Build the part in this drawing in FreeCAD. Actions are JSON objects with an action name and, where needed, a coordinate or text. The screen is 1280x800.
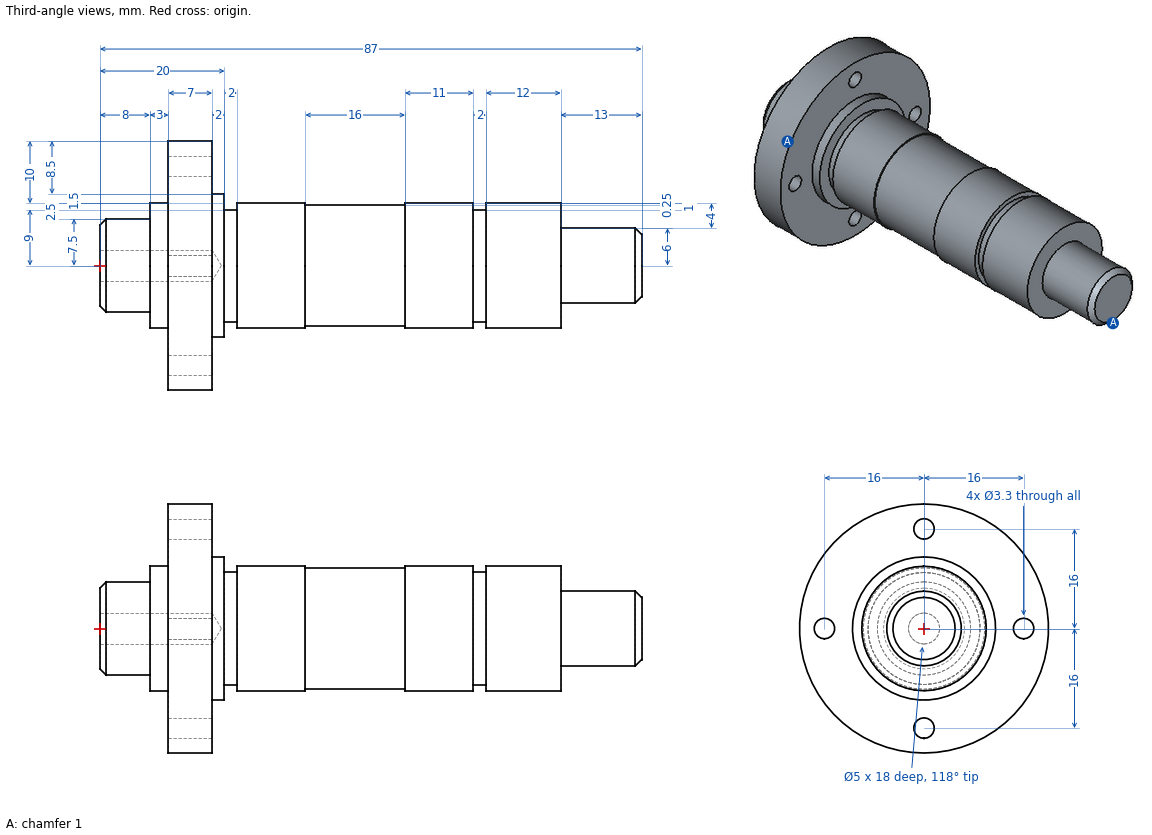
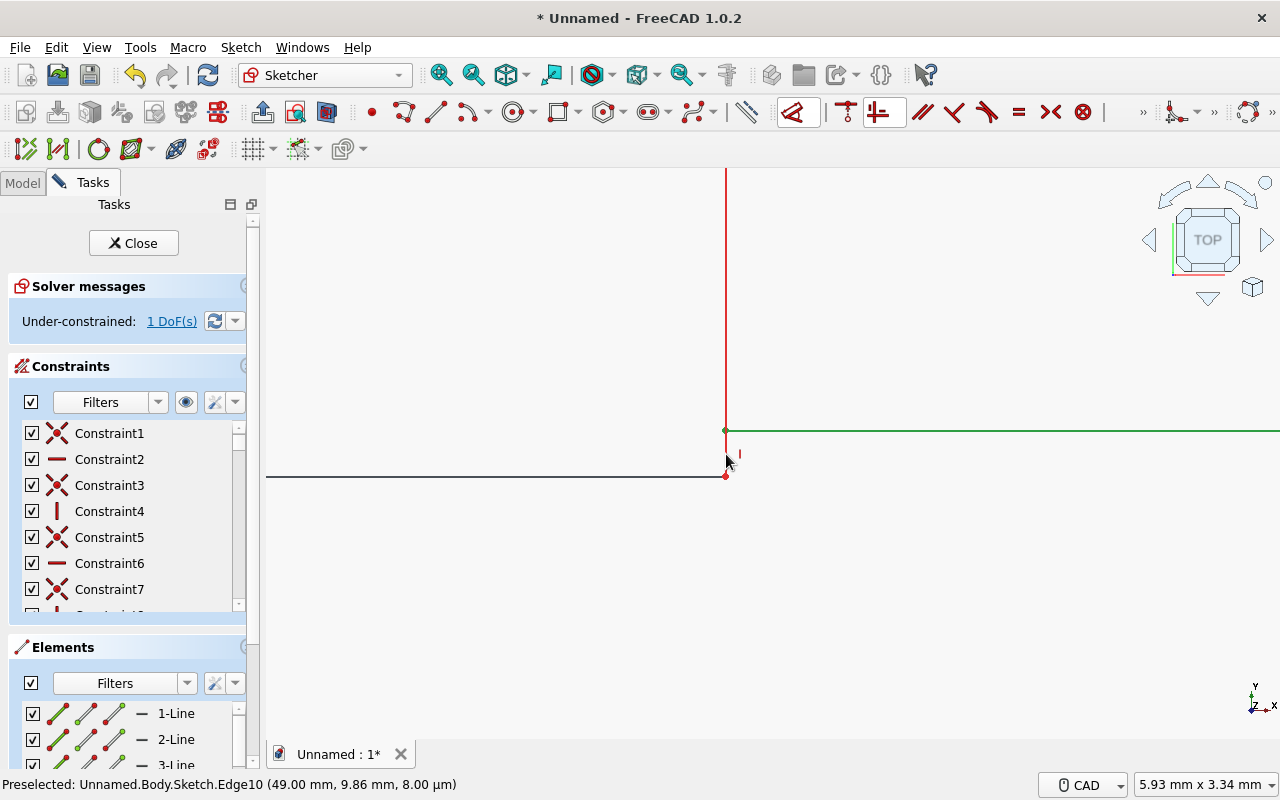
{"action": "left_click", "coordinate": [814, 112]}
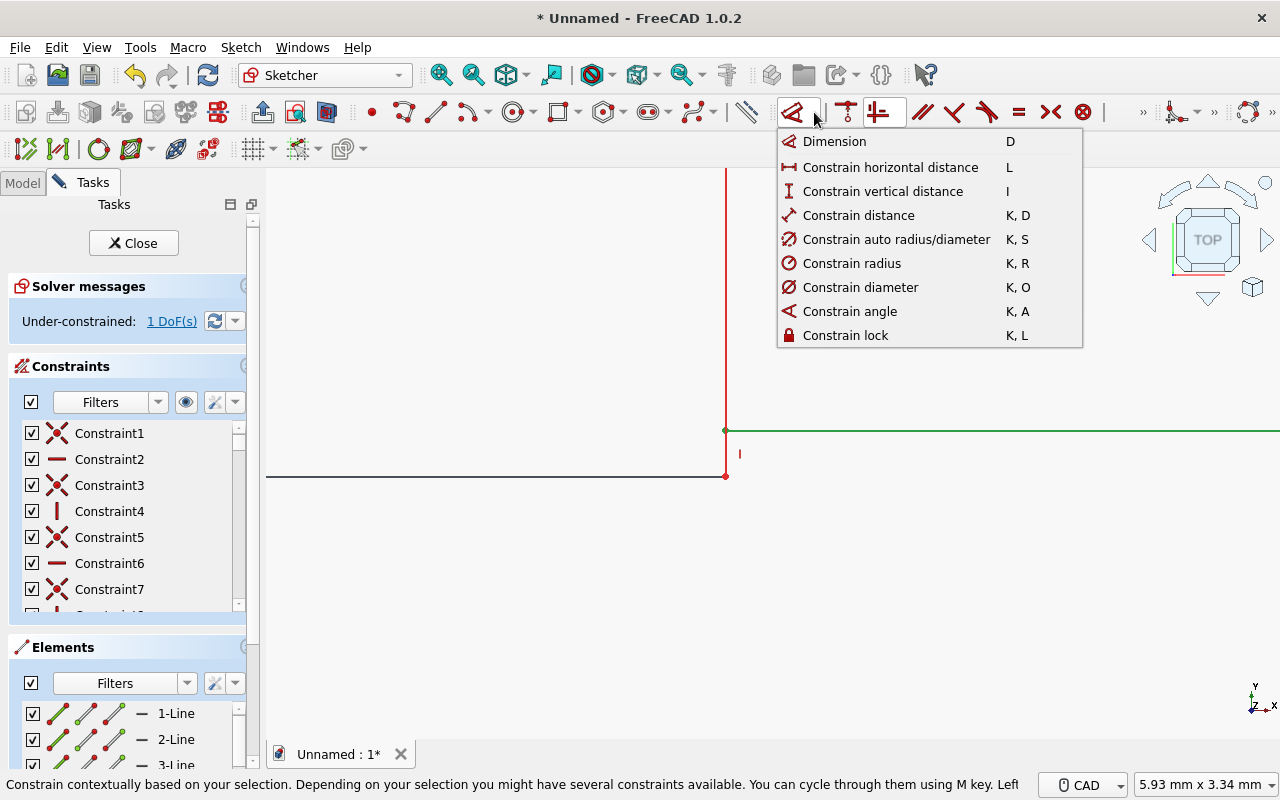
{"action": "left_click", "coordinate": [930, 191]}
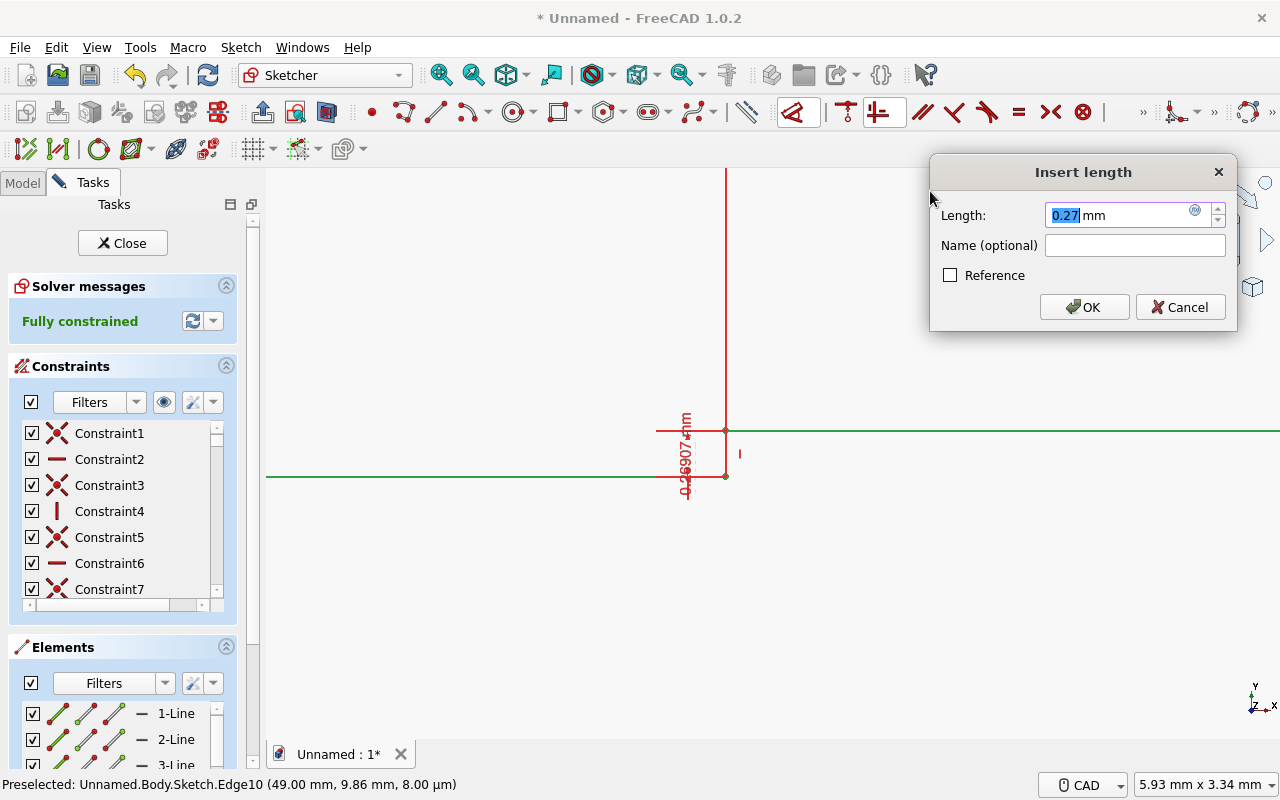
{"action": "type", "text": "0.25"}
{"action": "key", "text": "Return"}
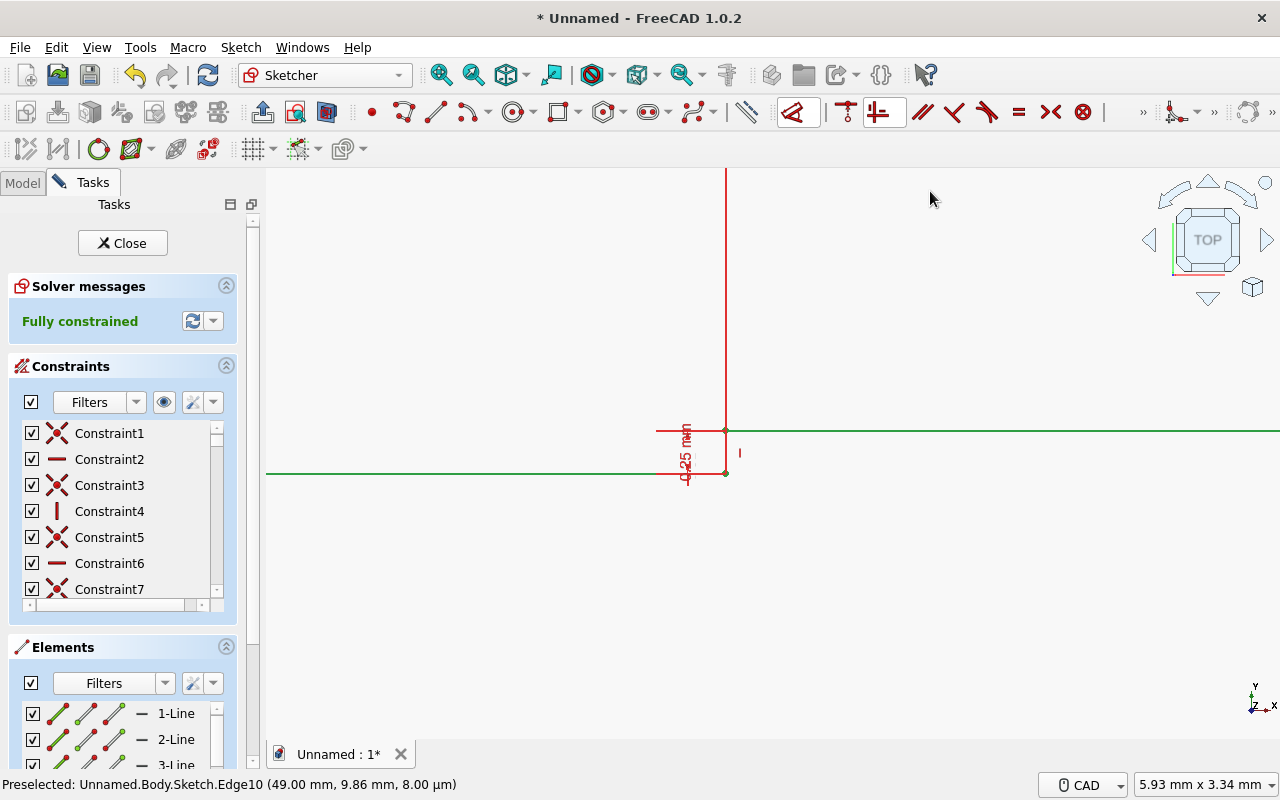
{"action": "left_click", "coordinate": [123, 243]}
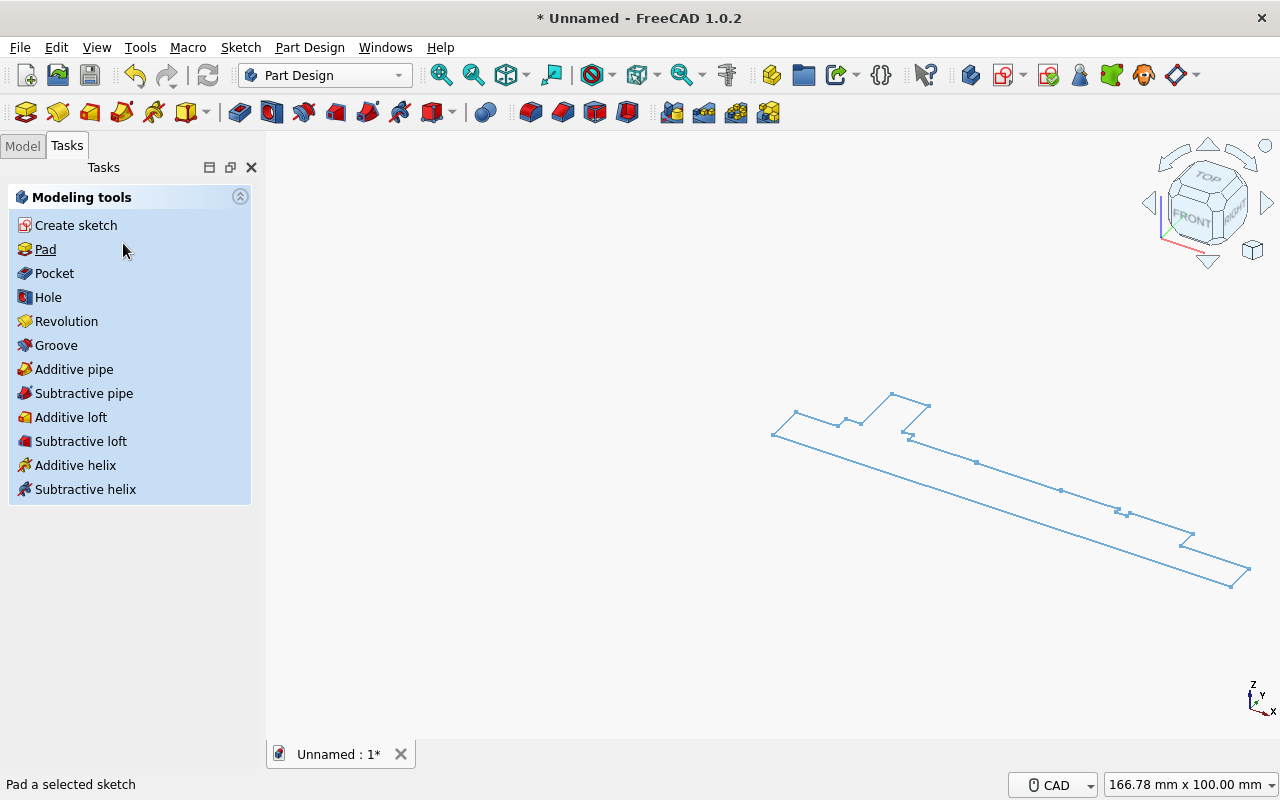
{"action": "left_click", "coordinate": [58, 112]}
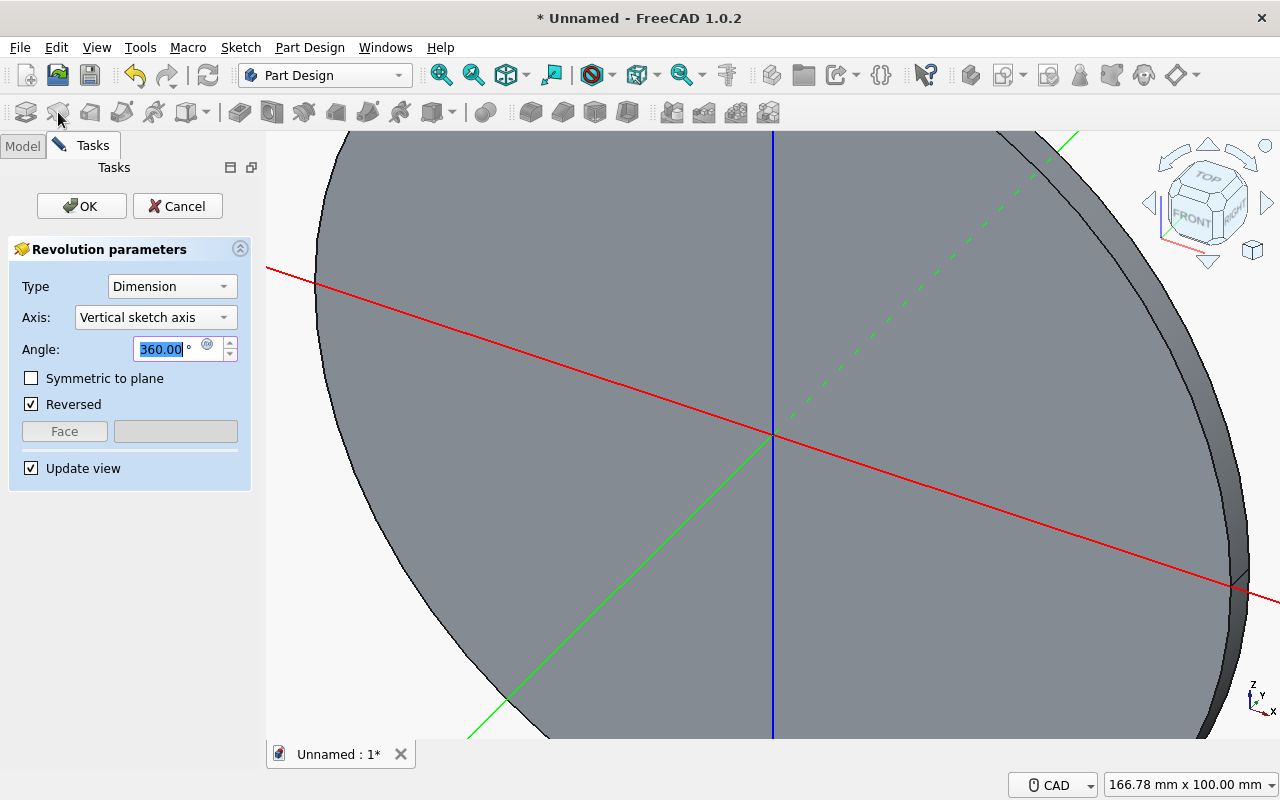
{"action": "left_click", "coordinate": [156, 318]}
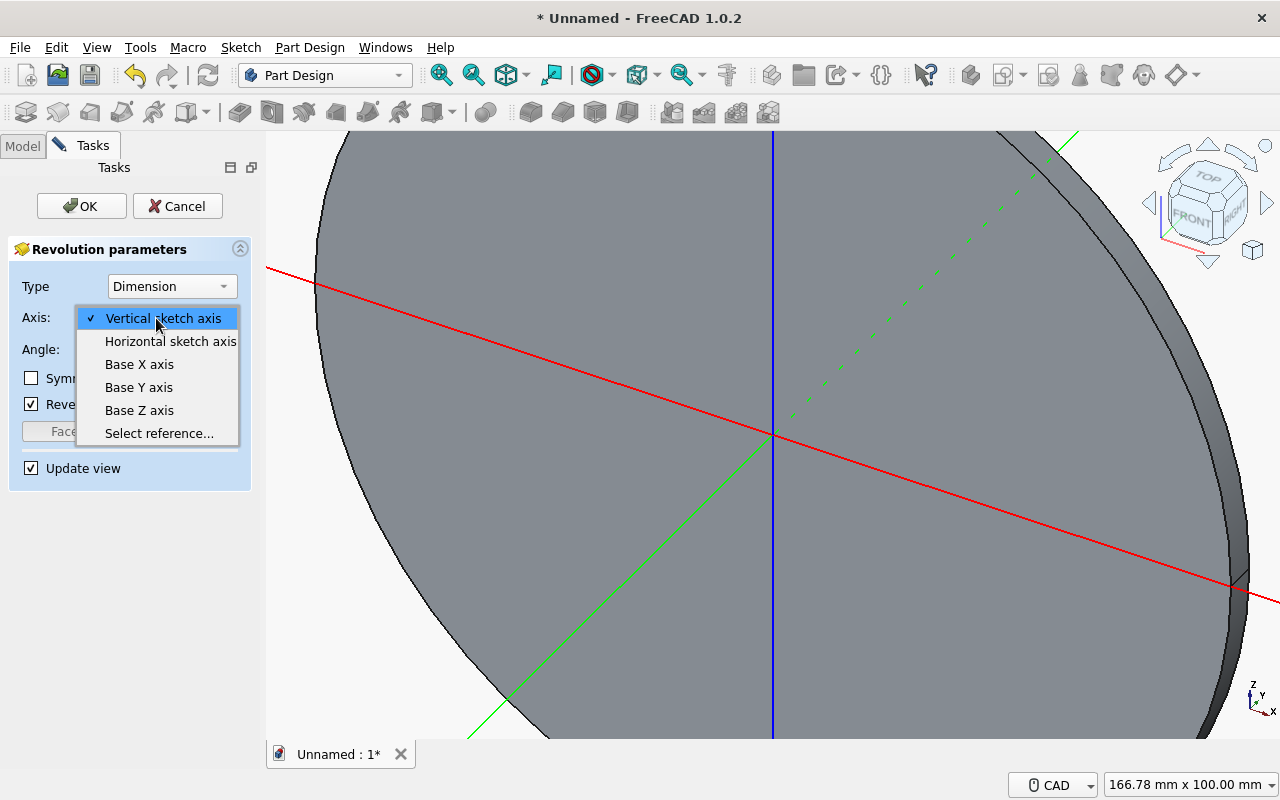
{"action": "left_click", "coordinate": [156, 342]}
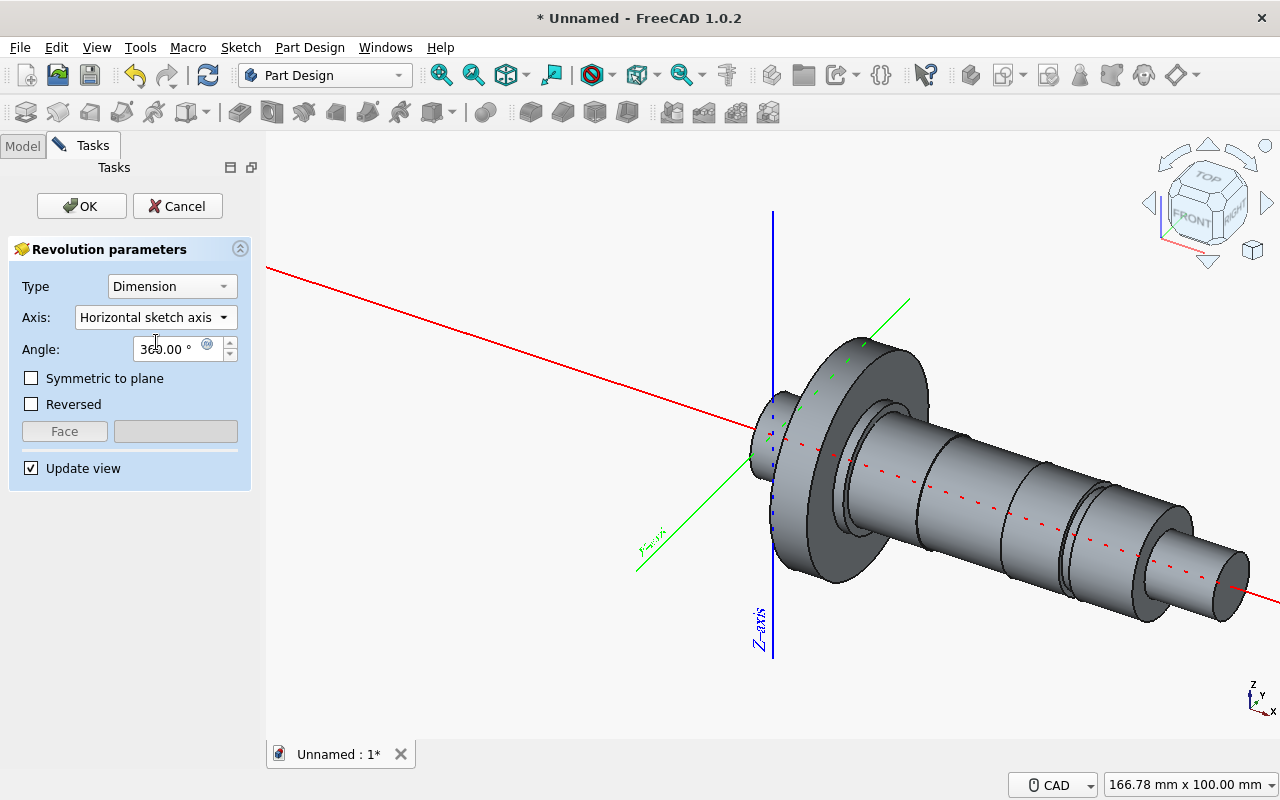
{"action": "left_click", "coordinate": [82, 206]}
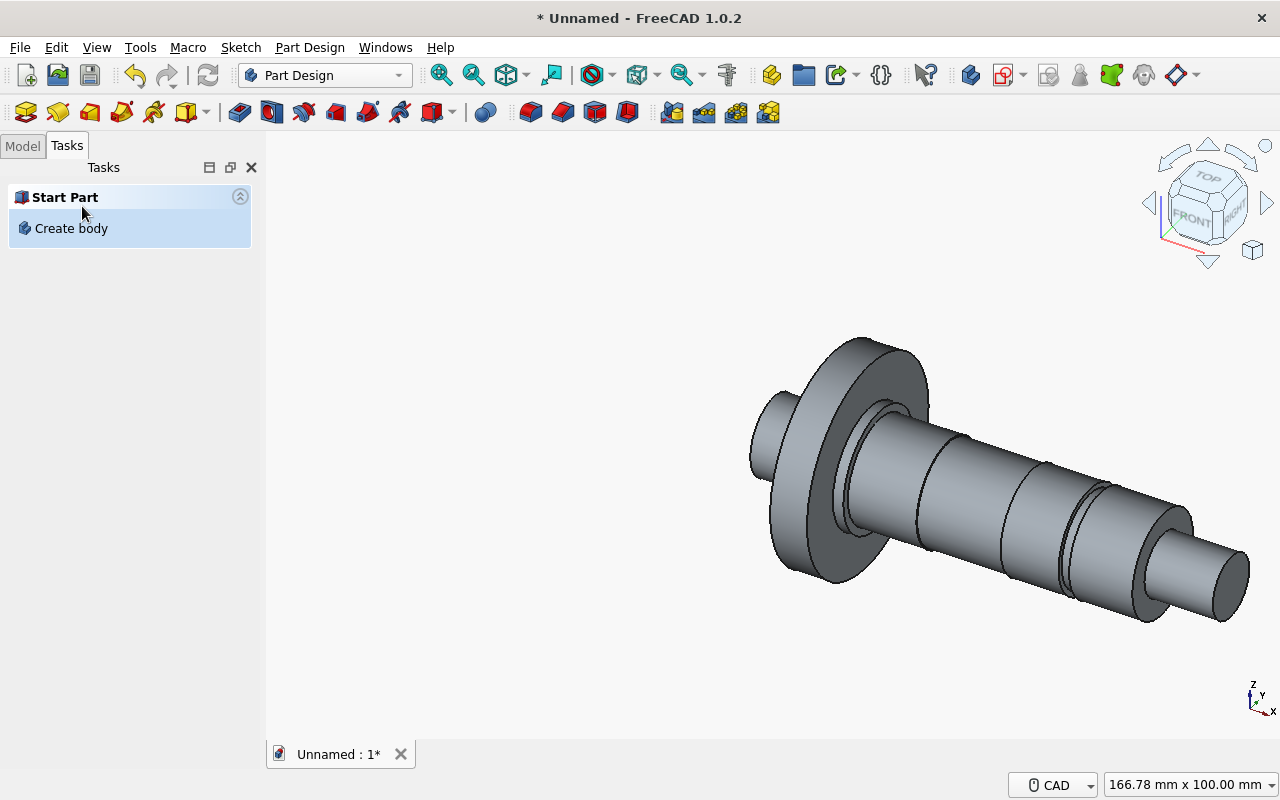
{"action": "left_click", "coordinate": [442, 76]}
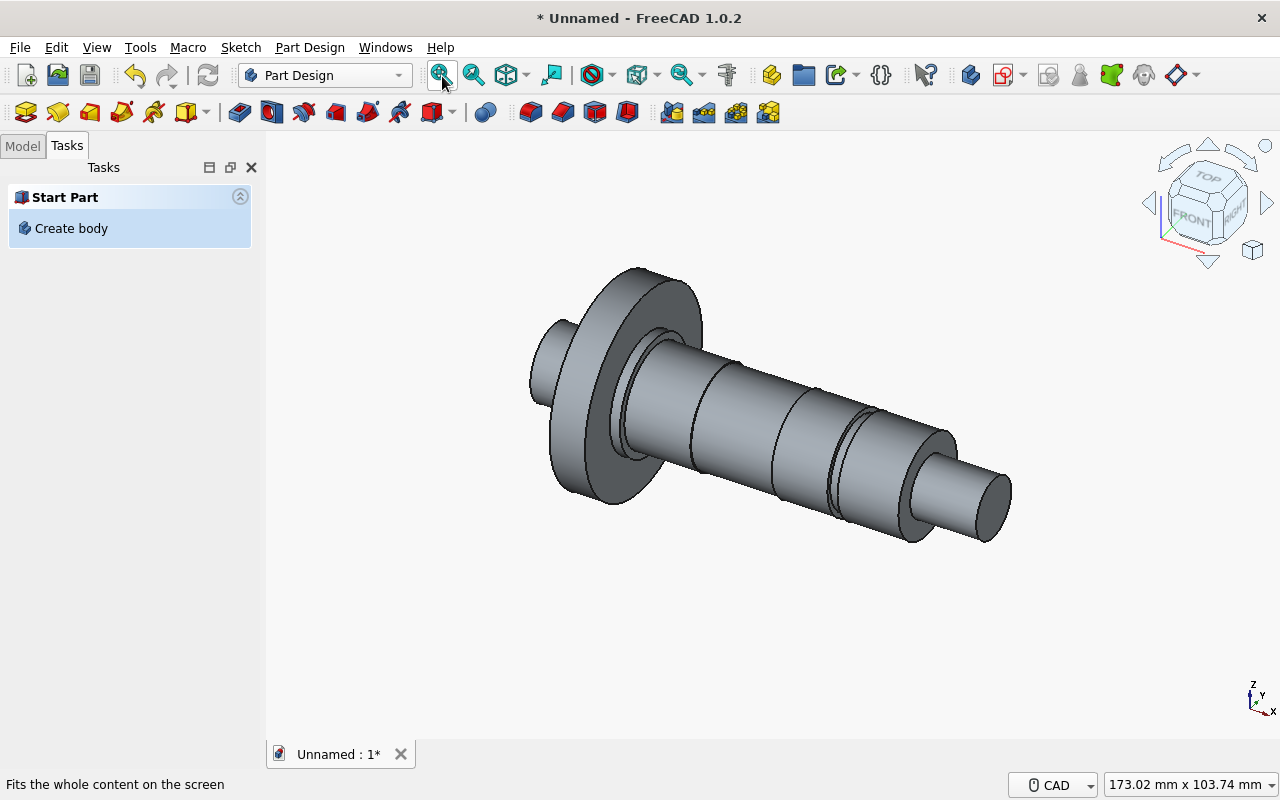
{"action": "key", "text": "6"}